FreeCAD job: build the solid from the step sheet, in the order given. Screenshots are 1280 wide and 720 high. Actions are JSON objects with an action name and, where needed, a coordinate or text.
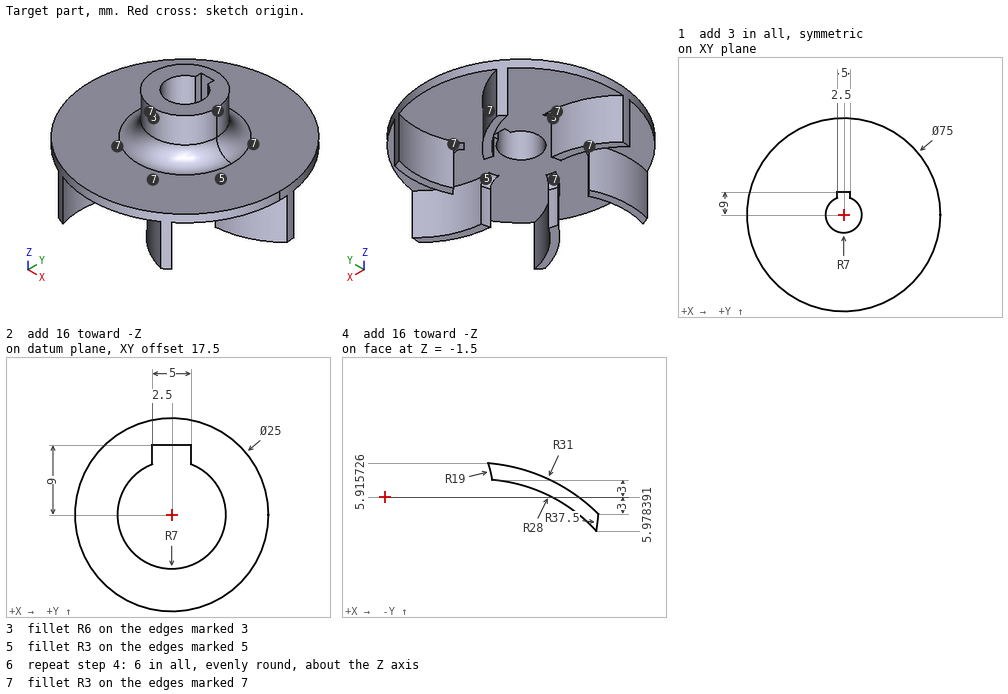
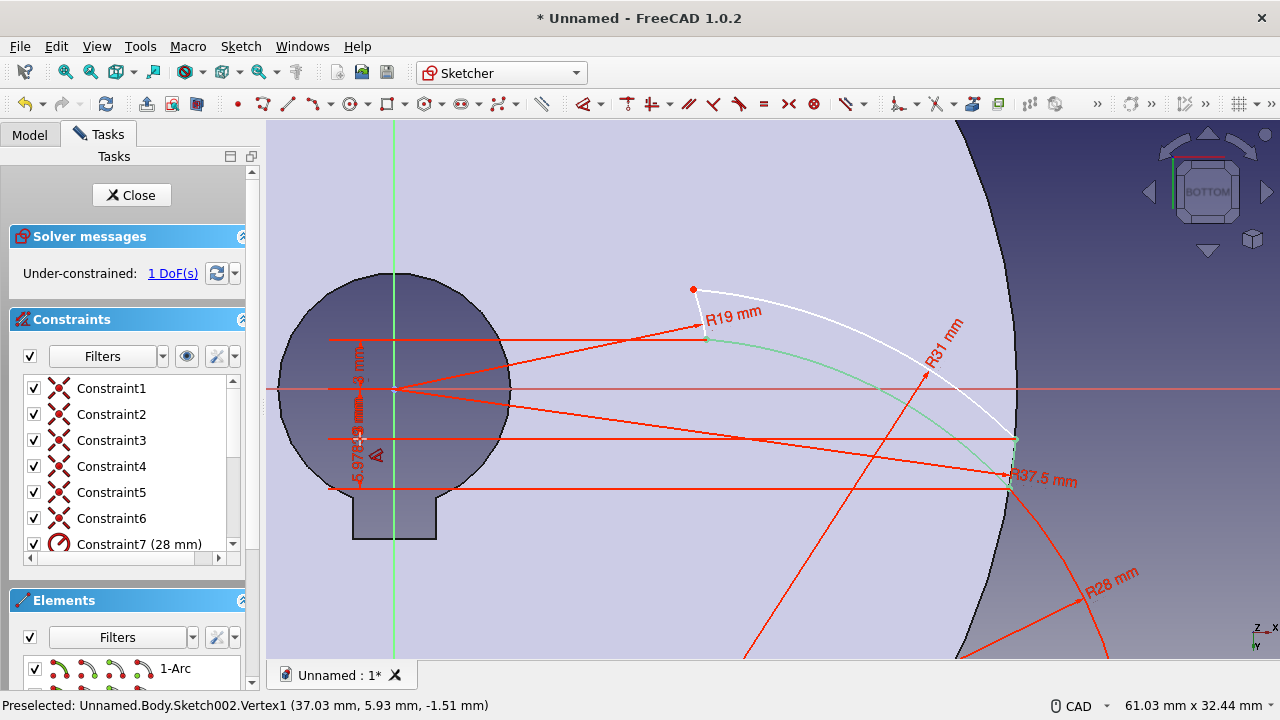
{"action": "left_click", "coordinate": [694, 290]}
{"action": "left_click", "coordinate": [360, 340]}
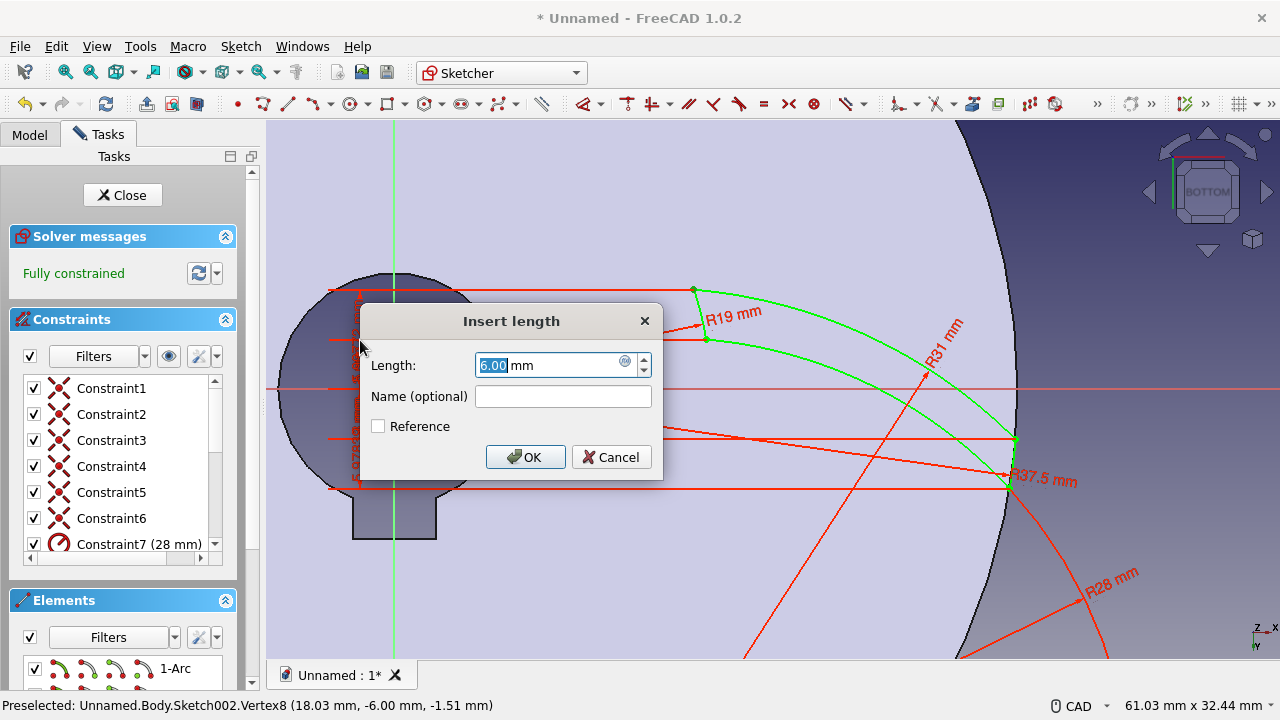
{"action": "type", "text": "5.915726"}
{"action": "key", "text": "Return"}
{"action": "key", "text": "Escape"}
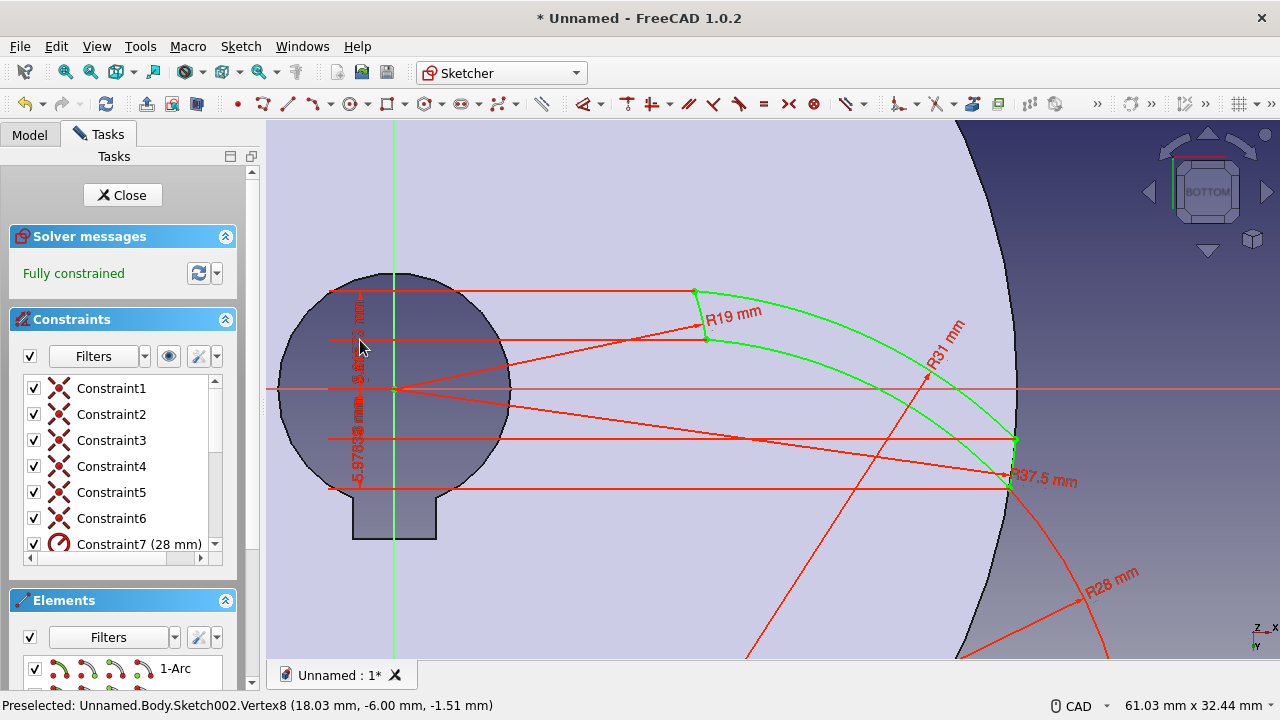
{"action": "left_click", "coordinate": [123, 195]}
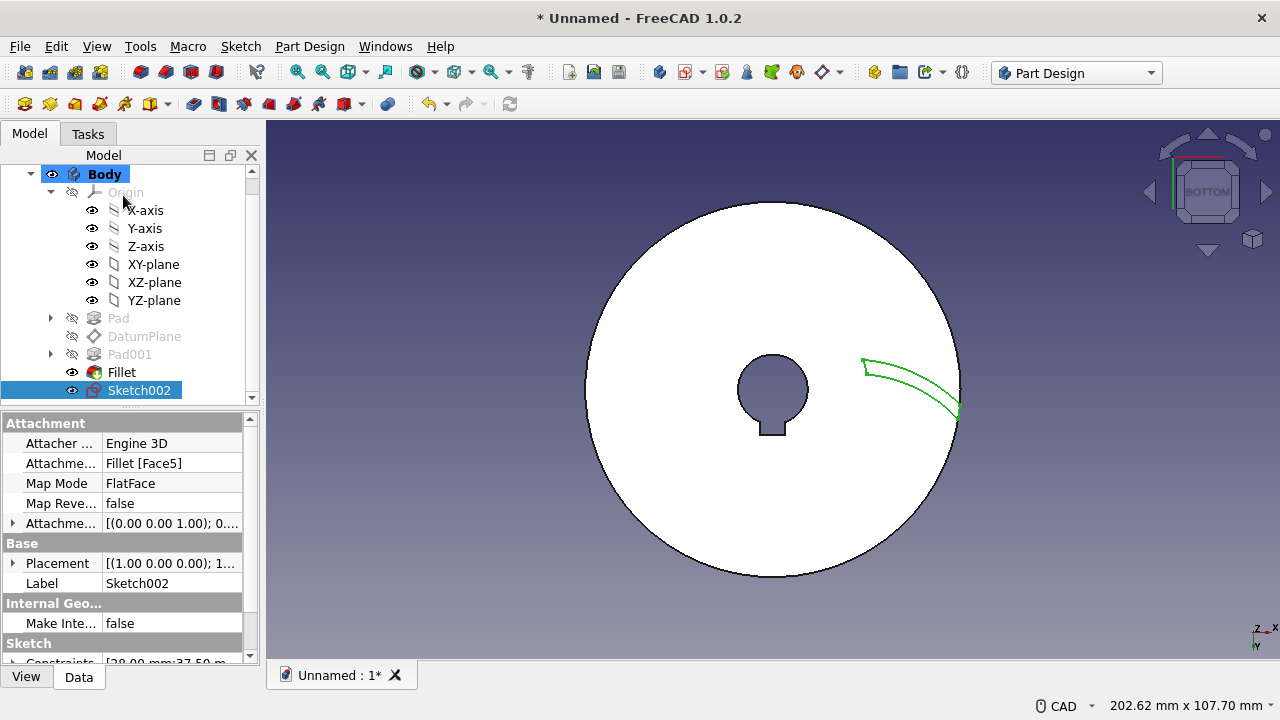
{"action": "left_click", "coordinate": [25, 104]}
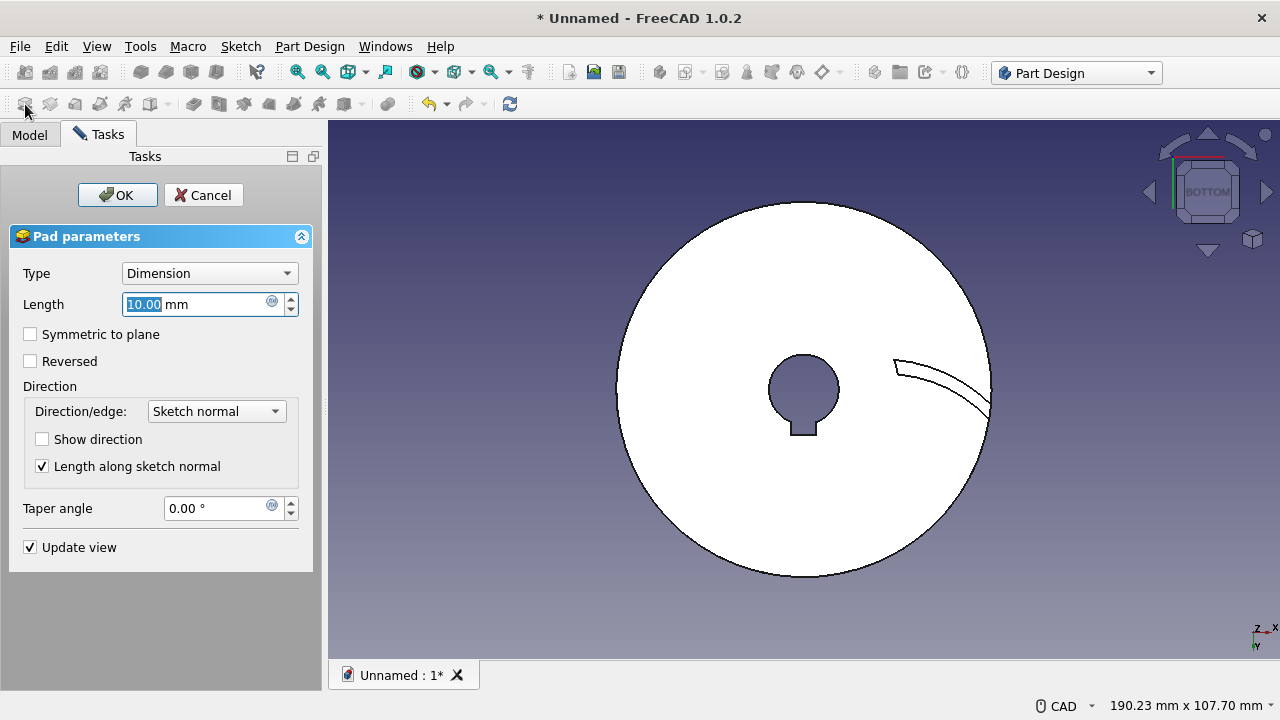
{"action": "type", "text": "16"}
{"action": "key", "text": "Tab"}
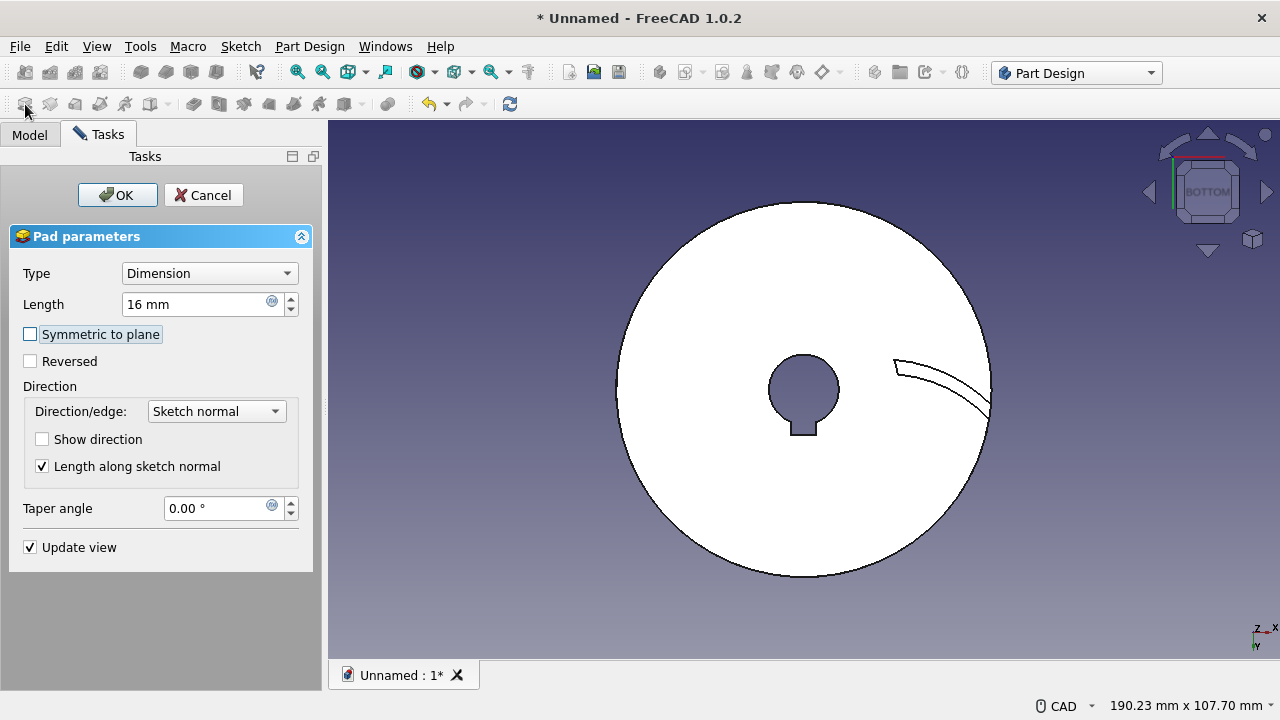
{"action": "left_click", "coordinate": [118, 195]}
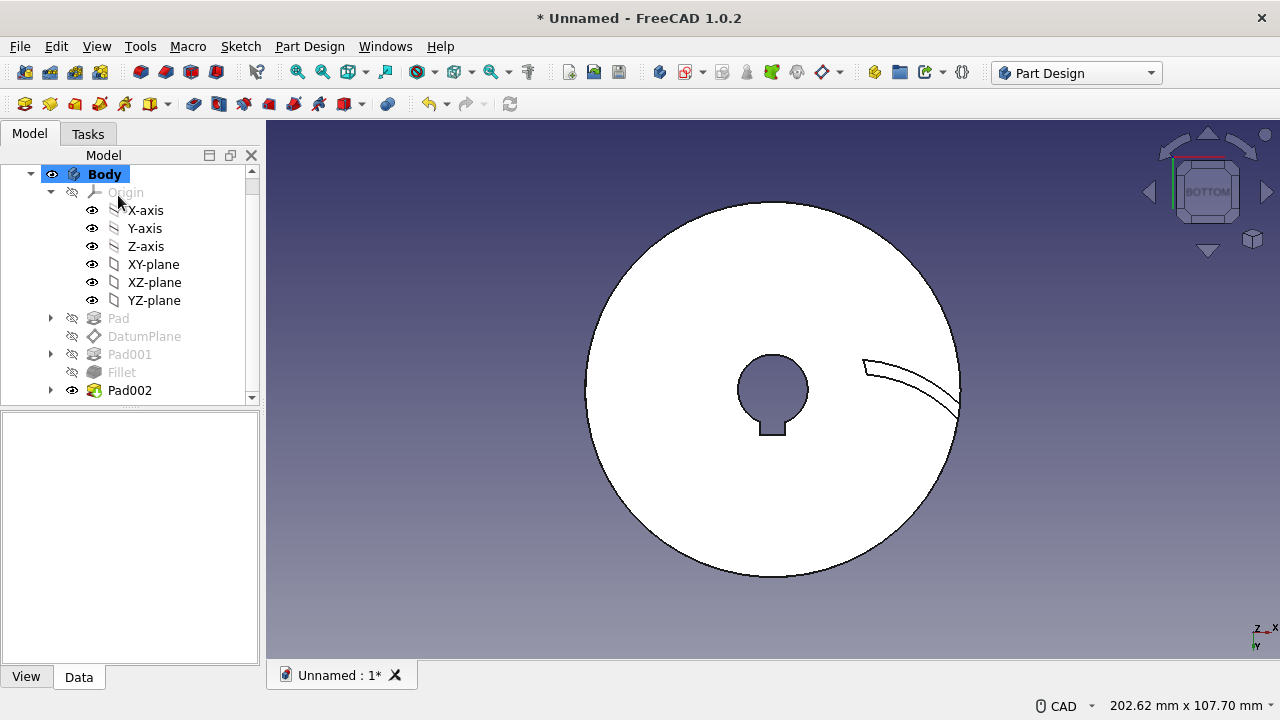
{"action": "scroll", "coordinate": [865, 366], "scroll_direction": "up", "scroll_amount": 5}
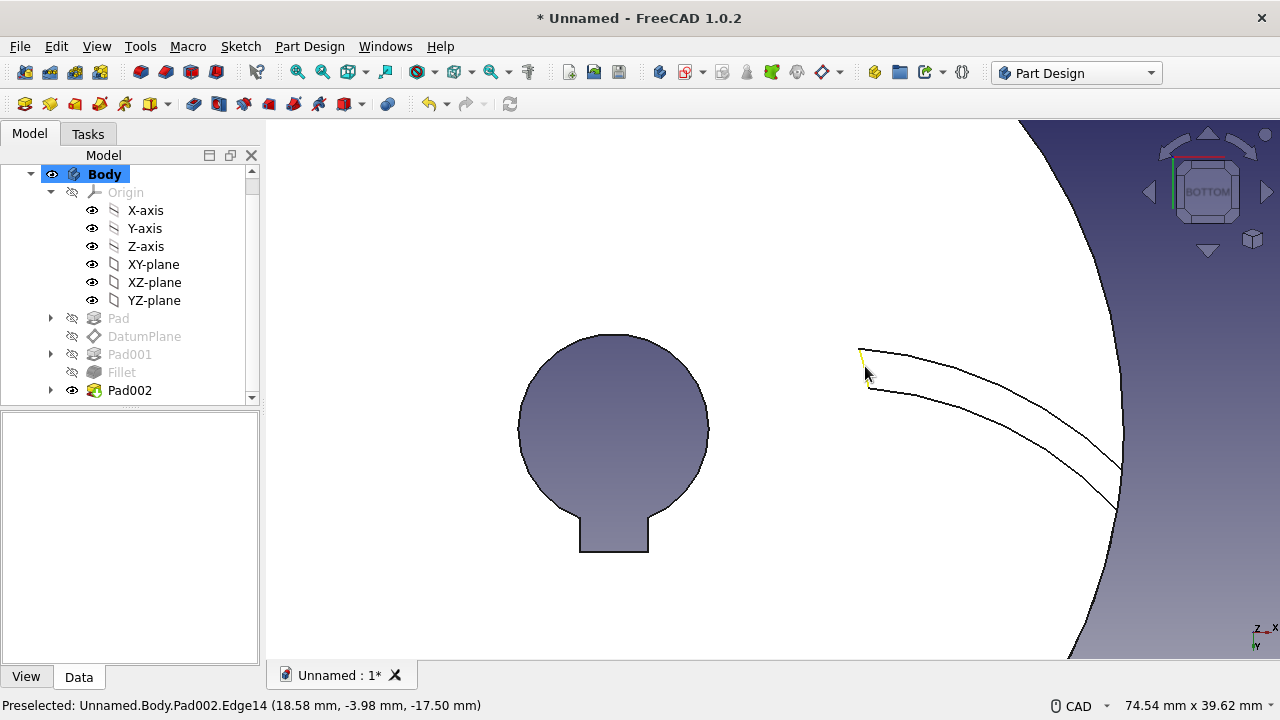
{"action": "left_click", "coordinate": [298, 72]}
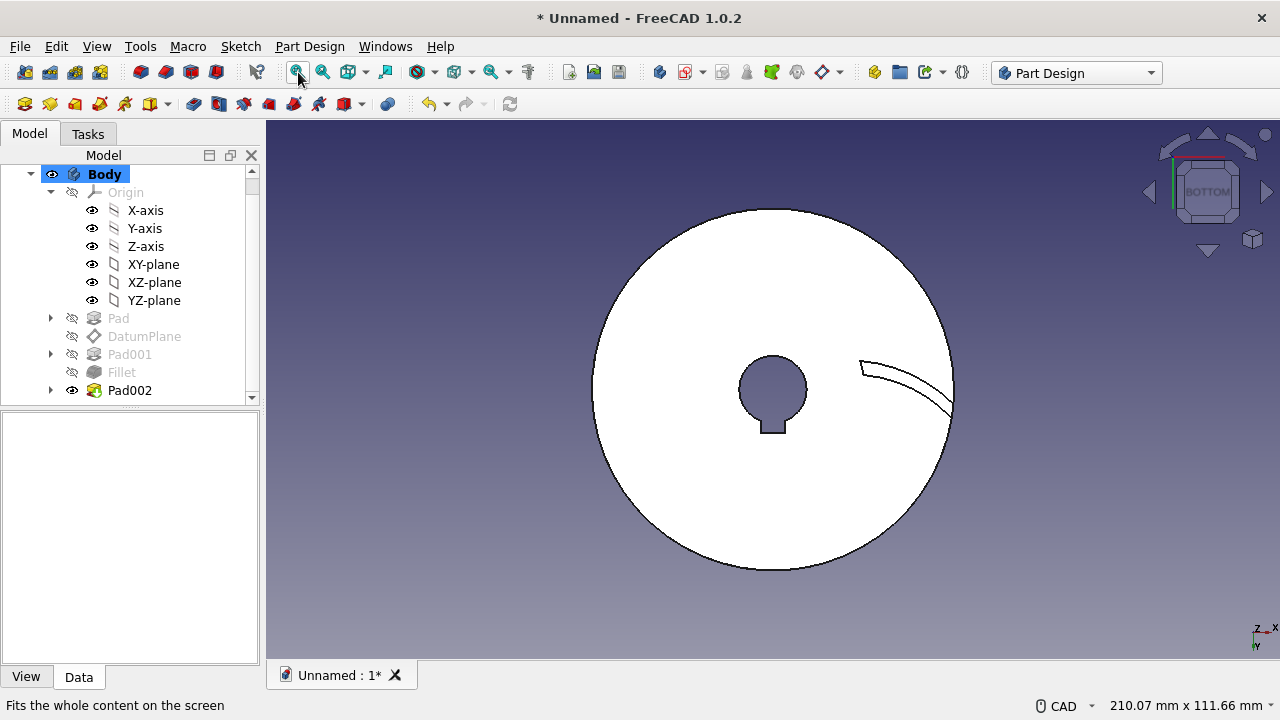
{"action": "key", "text": "0"}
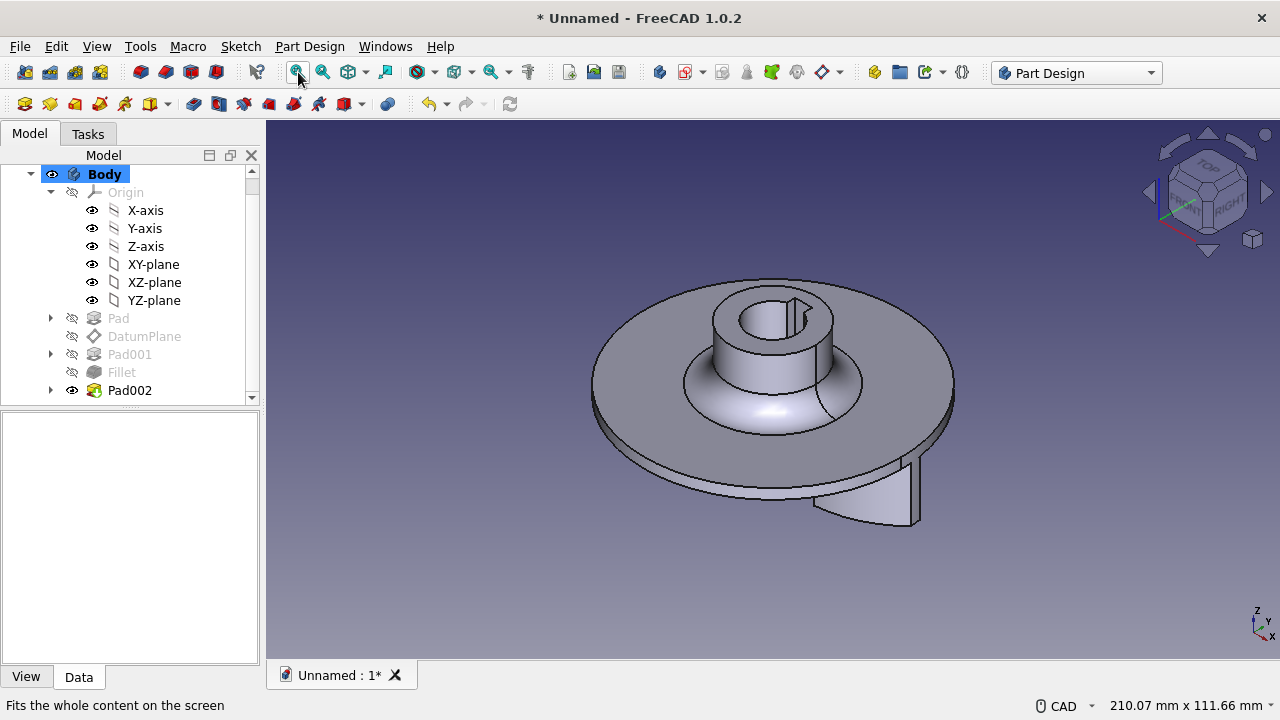
{"action": "scroll", "coordinate": [821, 440], "scroll_direction": "up", "scroll_amount": 6}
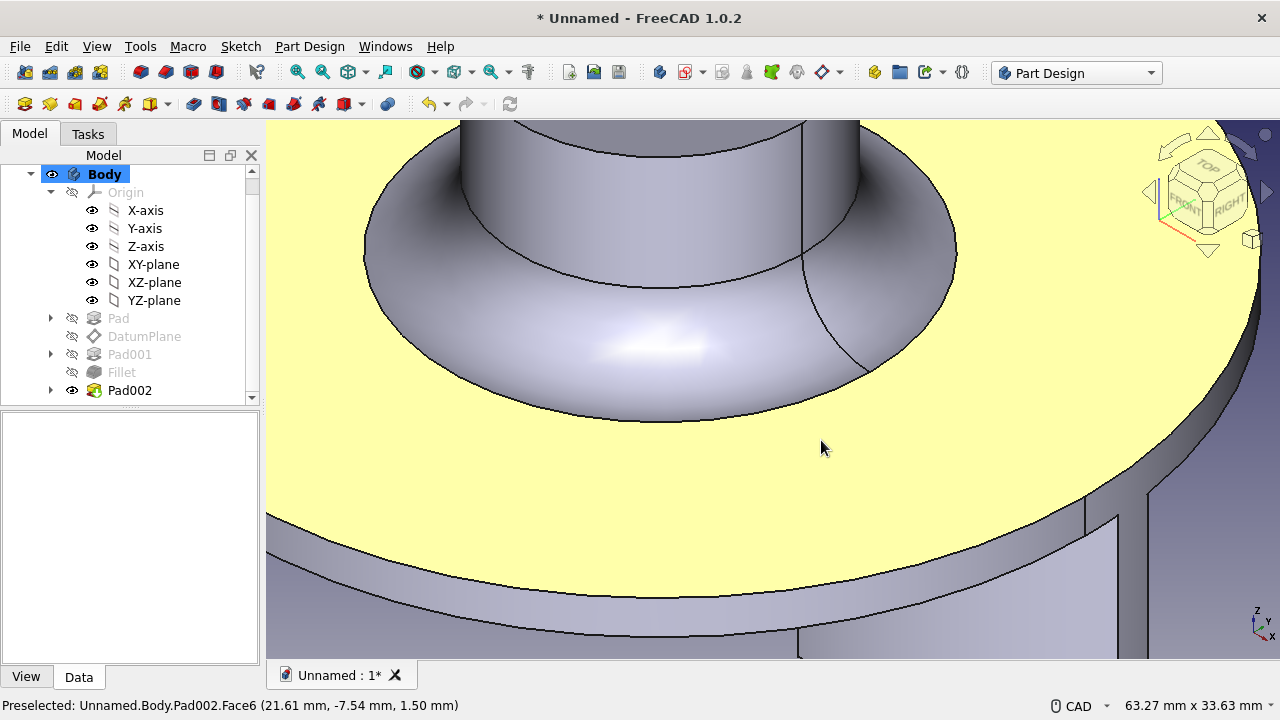
{"action": "left_click", "coordinate": [298, 72]}